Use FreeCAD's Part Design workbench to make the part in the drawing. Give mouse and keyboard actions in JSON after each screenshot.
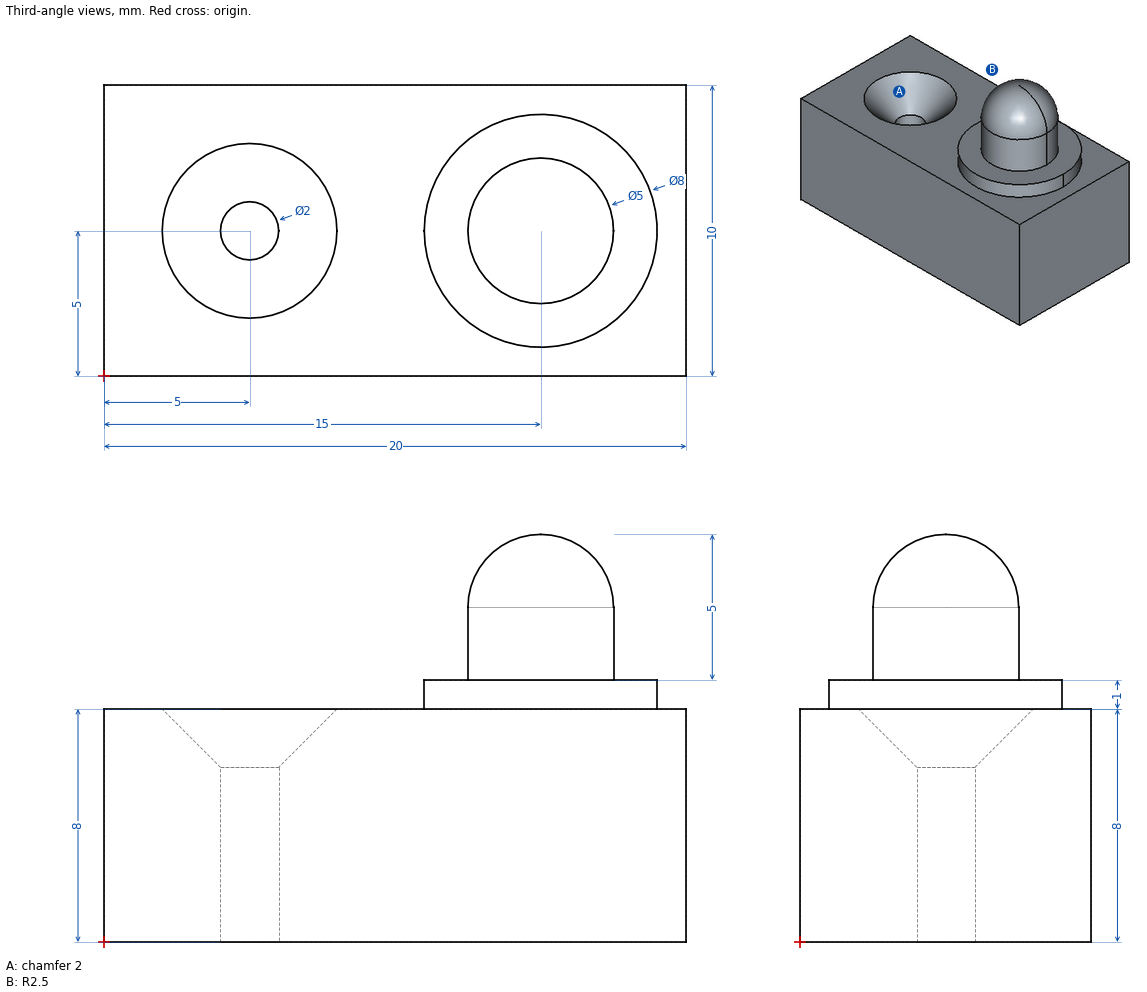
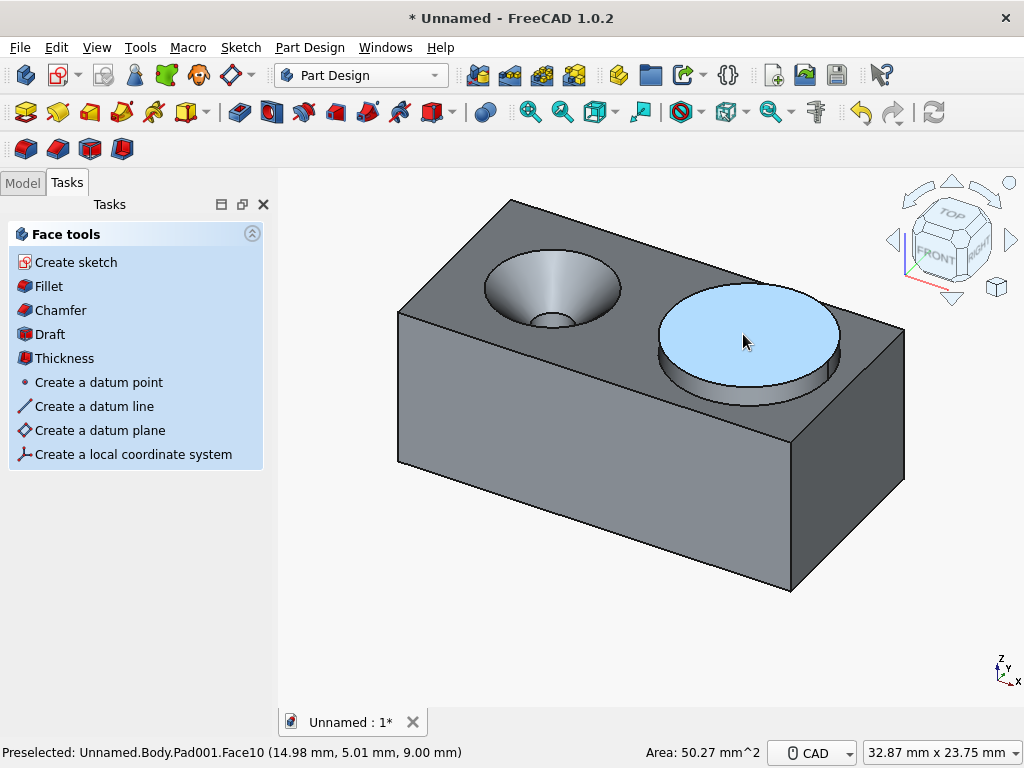
{"action": "left_click", "coordinate": [58, 76]}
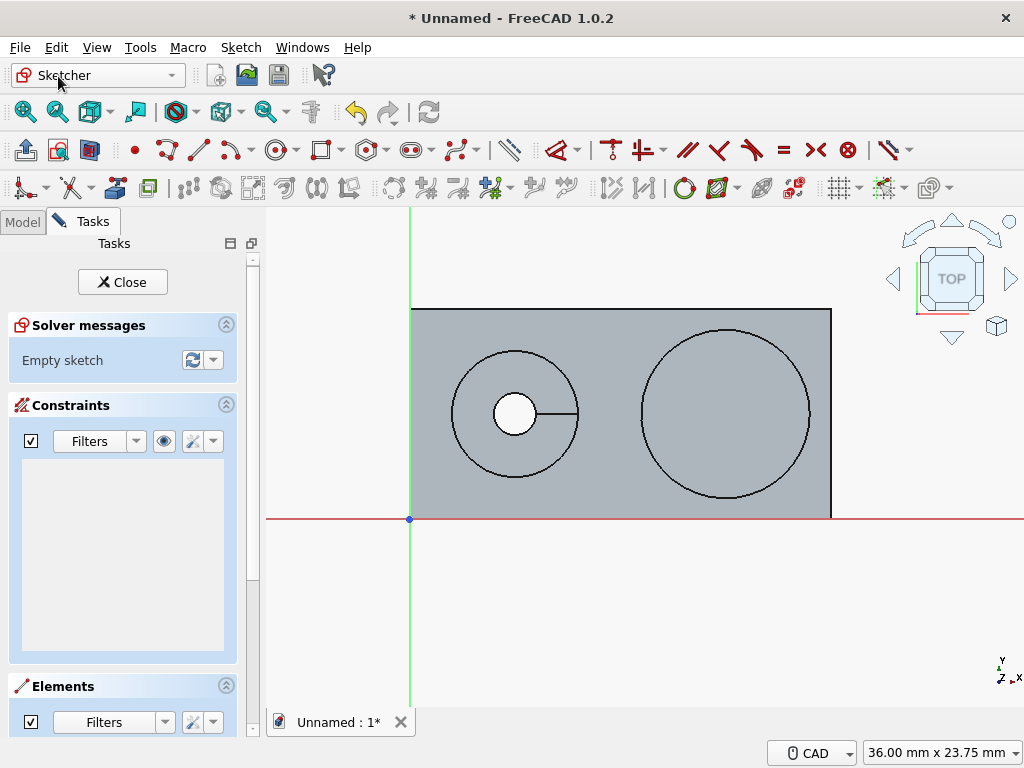
{"action": "scroll", "coordinate": [812, 389], "scroll_direction": "up", "scroll_amount": 5}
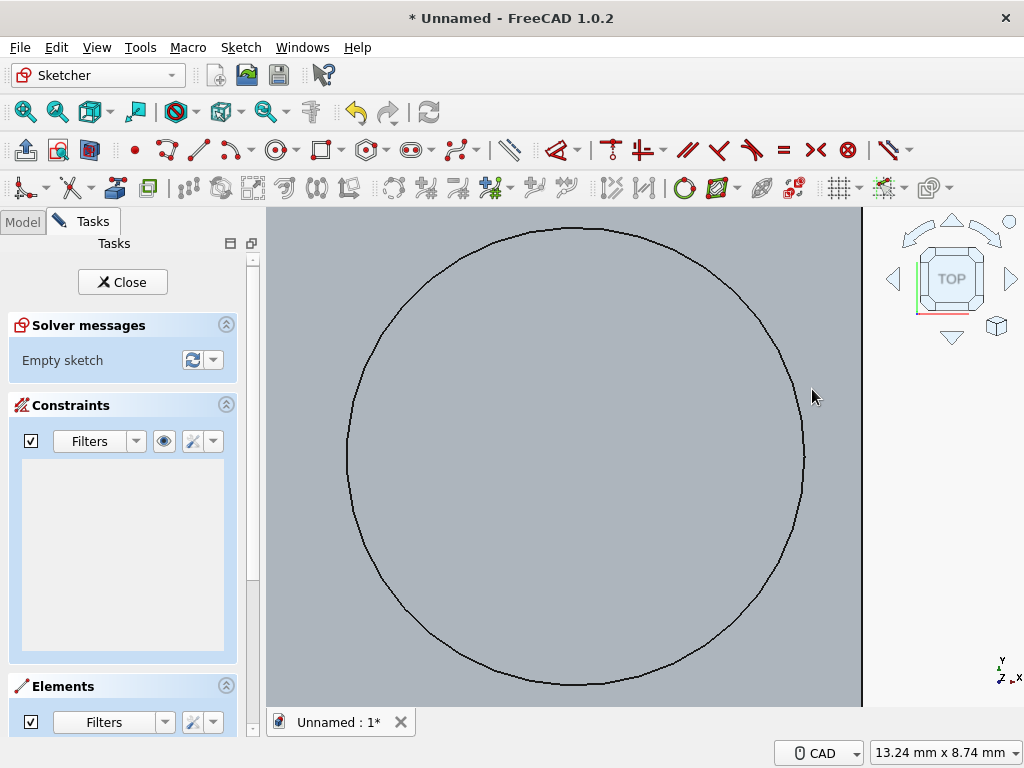
{"action": "left_click", "coordinate": [276, 150]}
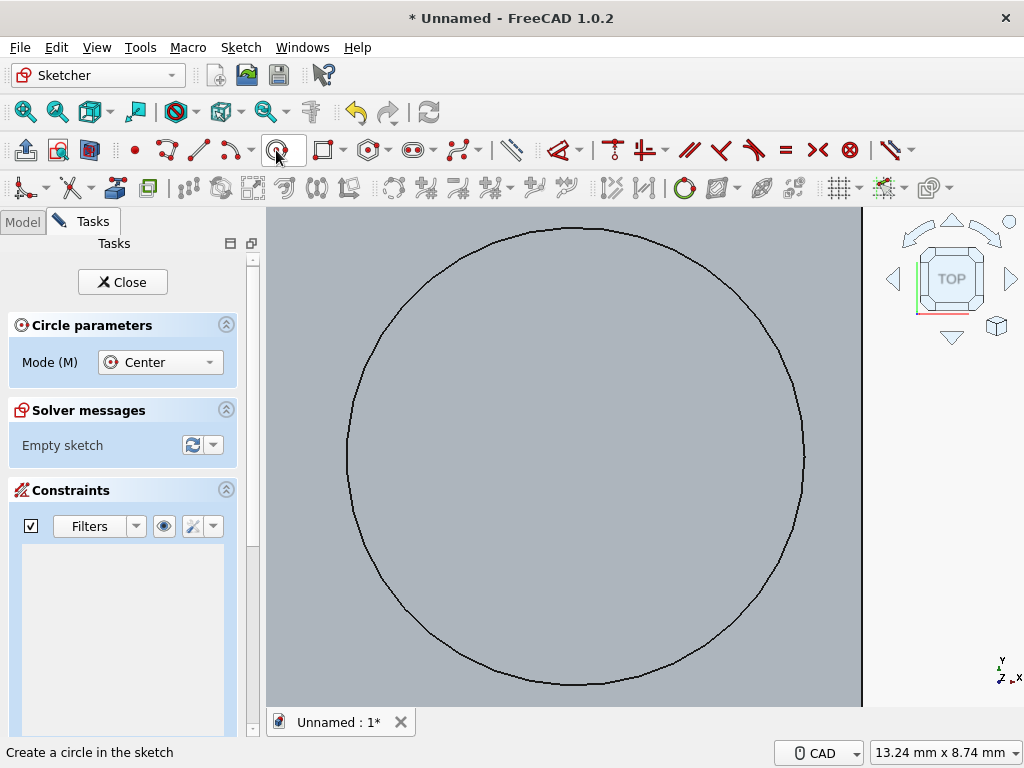
{"action": "left_click", "coordinate": [576, 457]}
{"action": "mouse_move", "coordinate": [677, 355]}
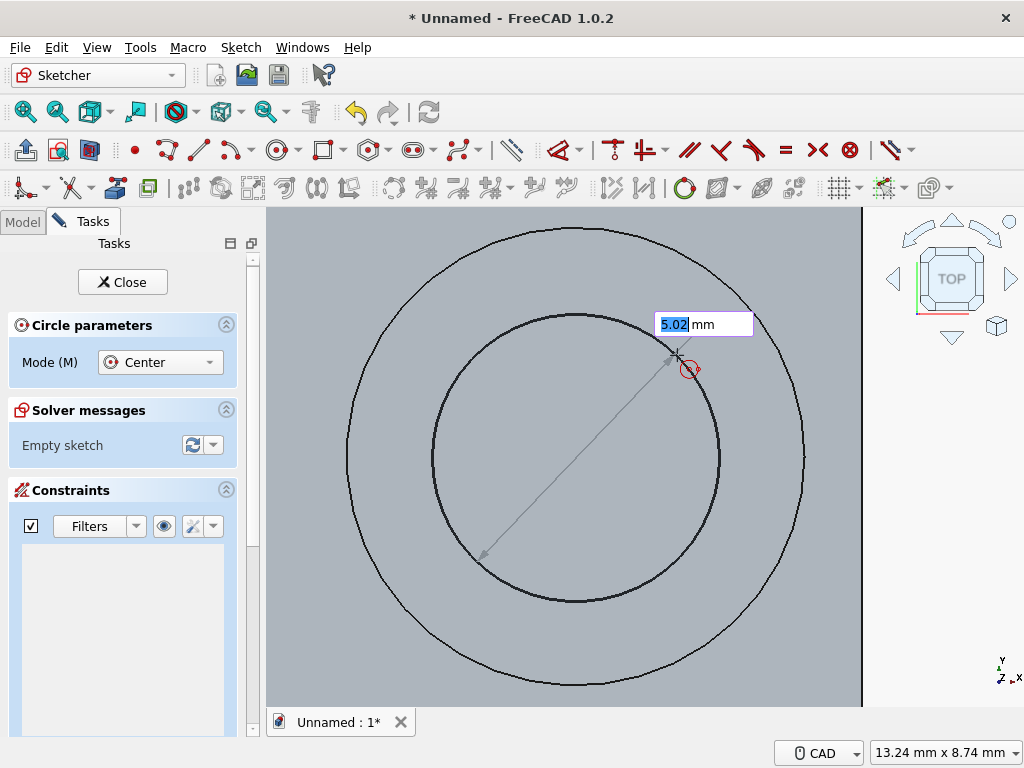
{"action": "type", "text": "5"}
{"action": "key", "text": "Return"}
{"action": "key", "text": "Escape"}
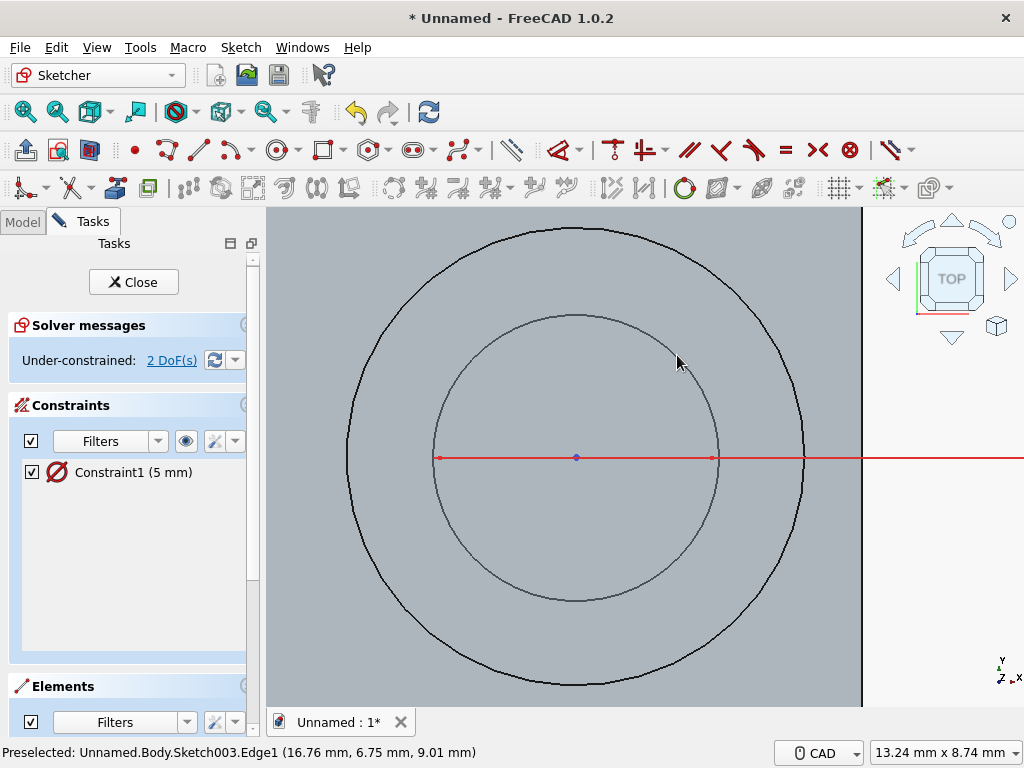
{"action": "left_click", "coordinate": [558, 150]}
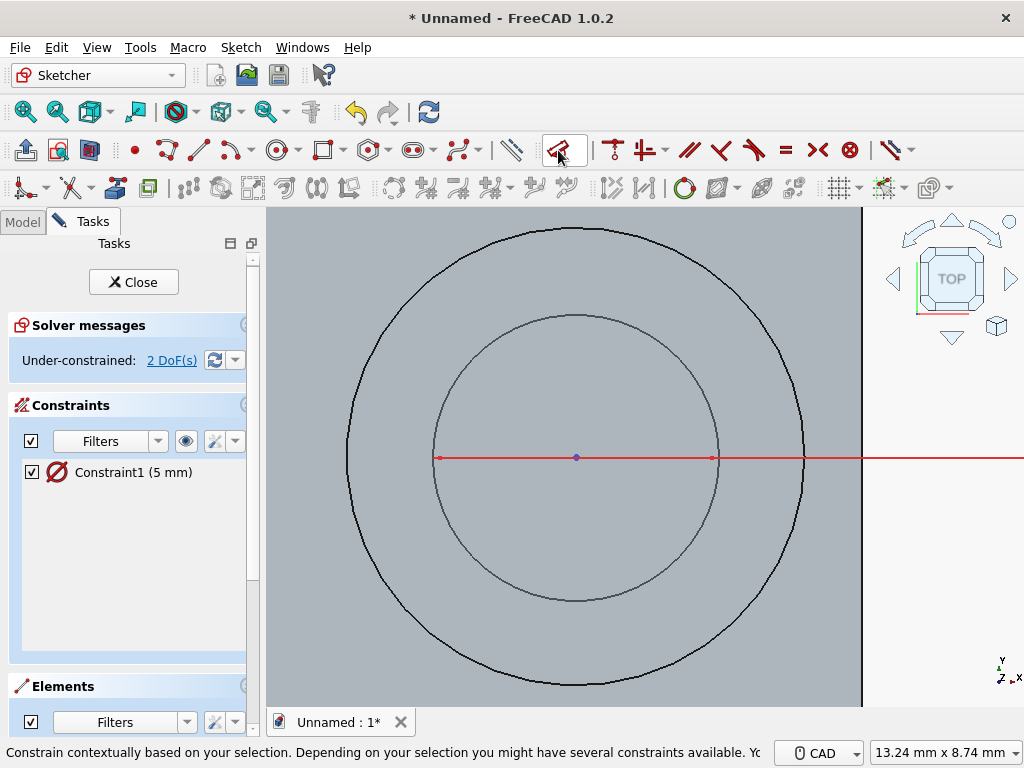
{"action": "left_click", "coordinate": [576, 458]}
{"action": "left_click", "coordinate": [610, 569]}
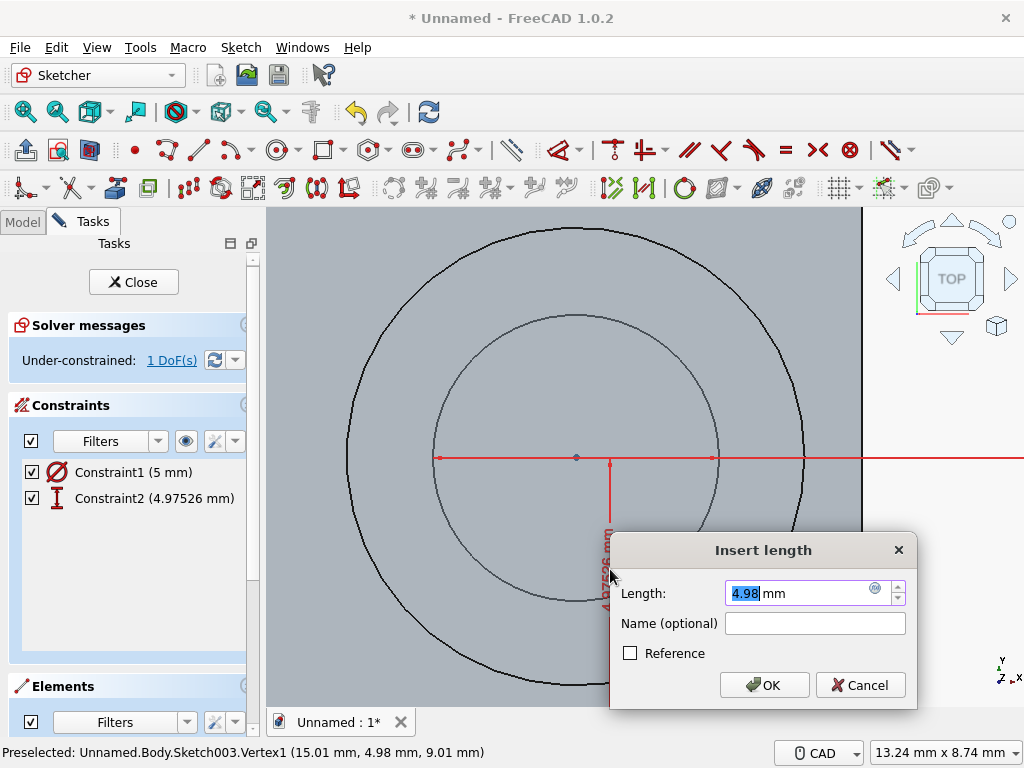
{"action": "type", "text": "5"}
{"action": "key", "text": "Return"}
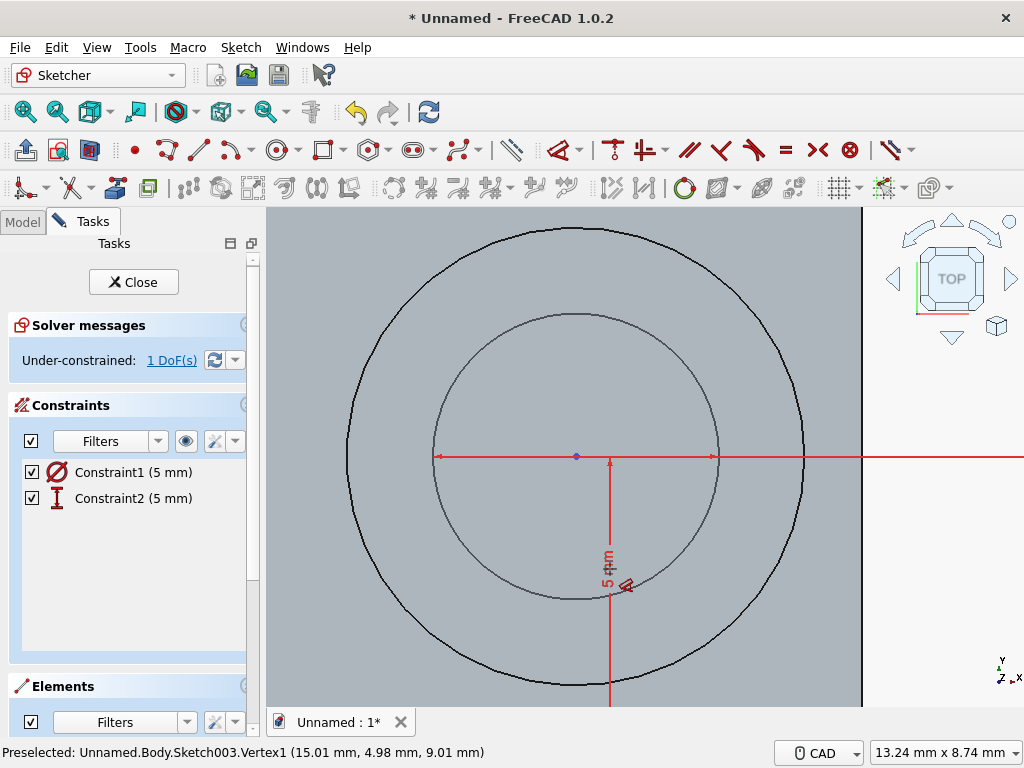
{"action": "left_click", "coordinate": [576, 457]}
{"action": "left_click", "coordinate": [370, 423]}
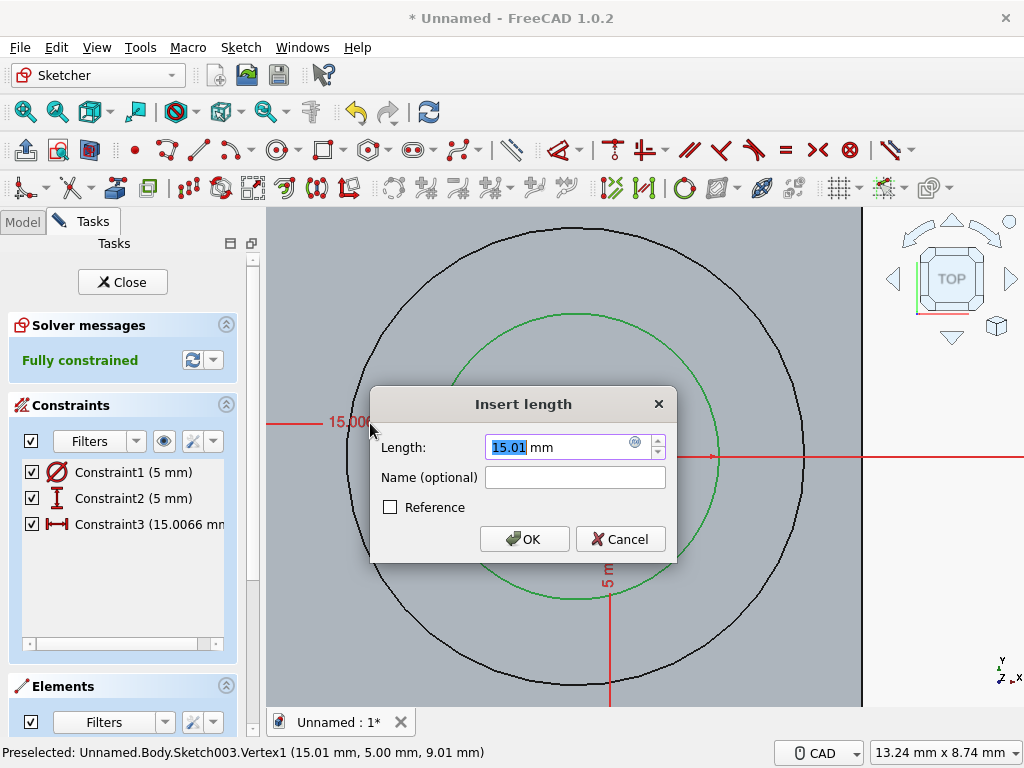
{"action": "type", "text": "15"}
{"action": "key", "text": "Return"}
{"action": "key", "text": "Escape"}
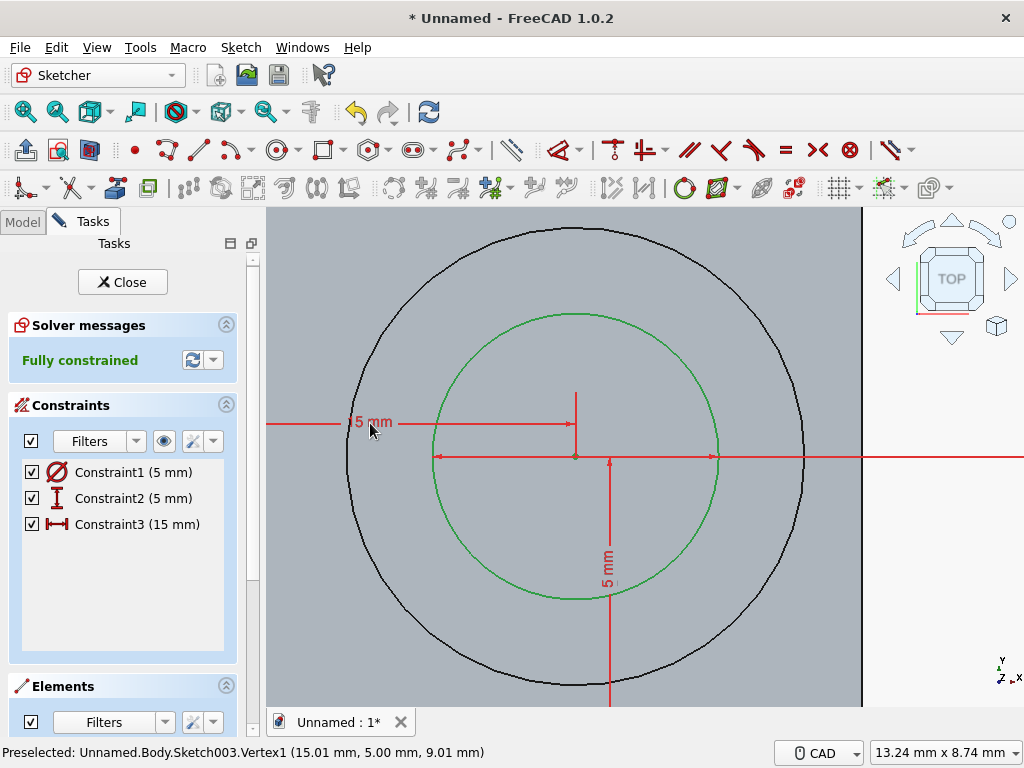
{"action": "left_click", "coordinate": [123, 282]}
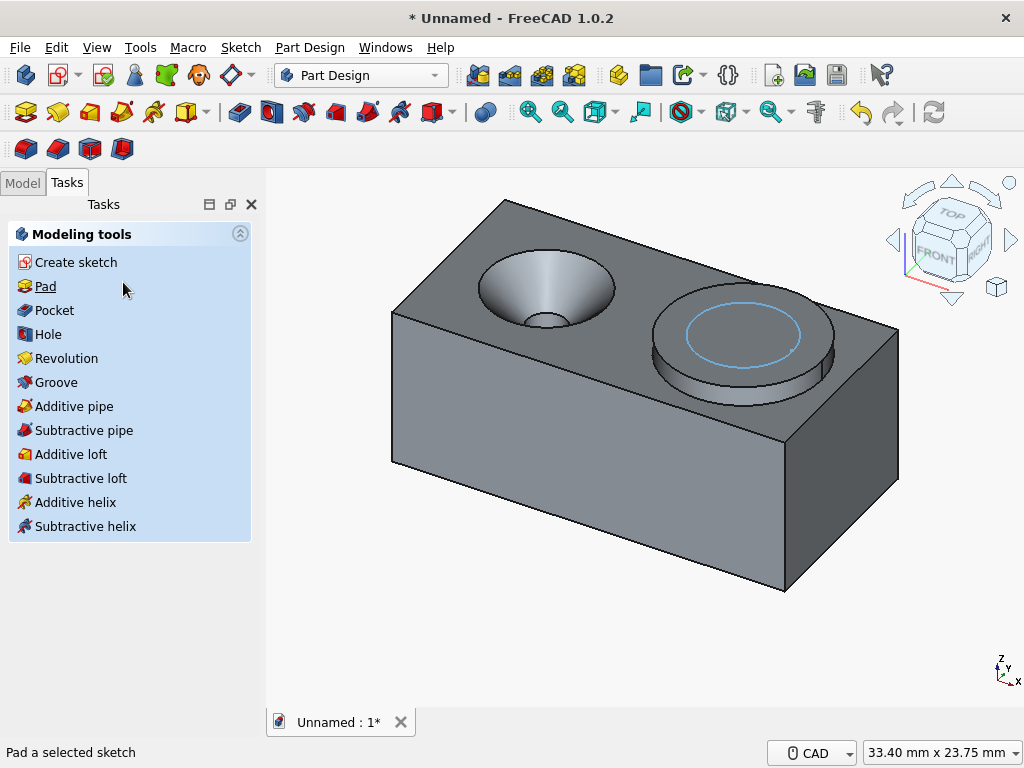
{"action": "left_click", "coordinate": [26, 112]}